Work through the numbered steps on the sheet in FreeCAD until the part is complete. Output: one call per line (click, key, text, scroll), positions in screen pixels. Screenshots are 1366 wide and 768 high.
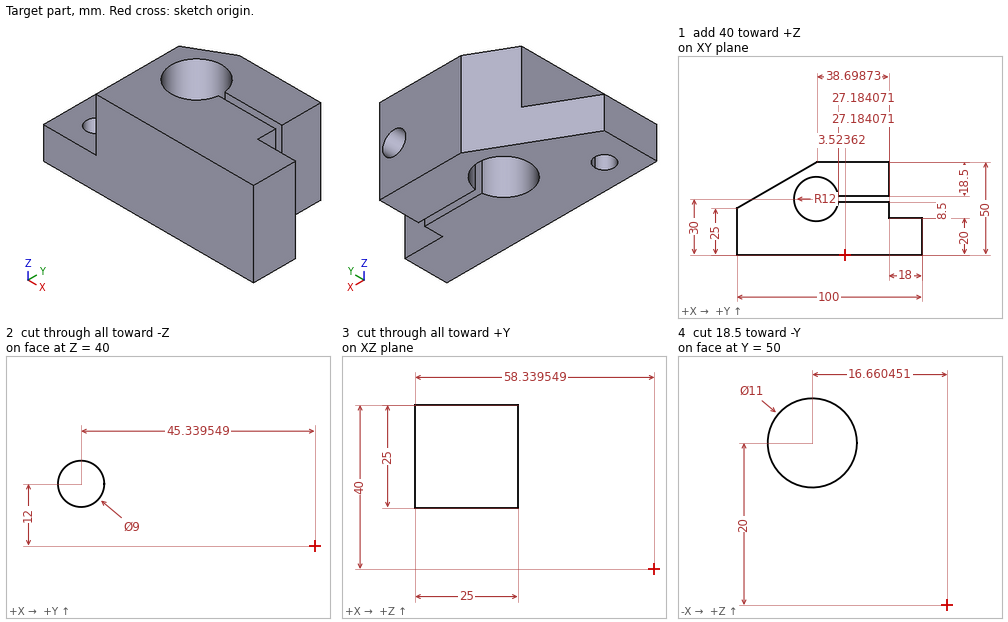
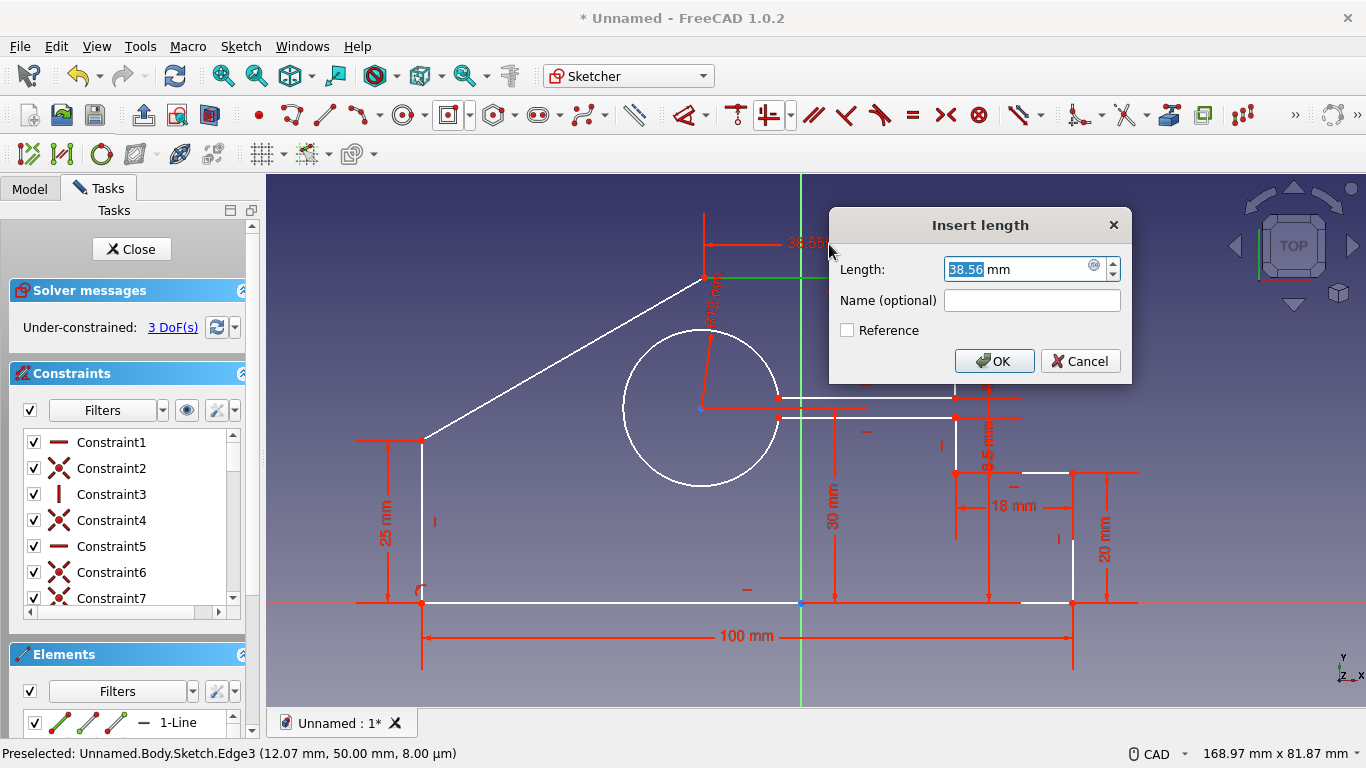
text(38.69873)
key(Return)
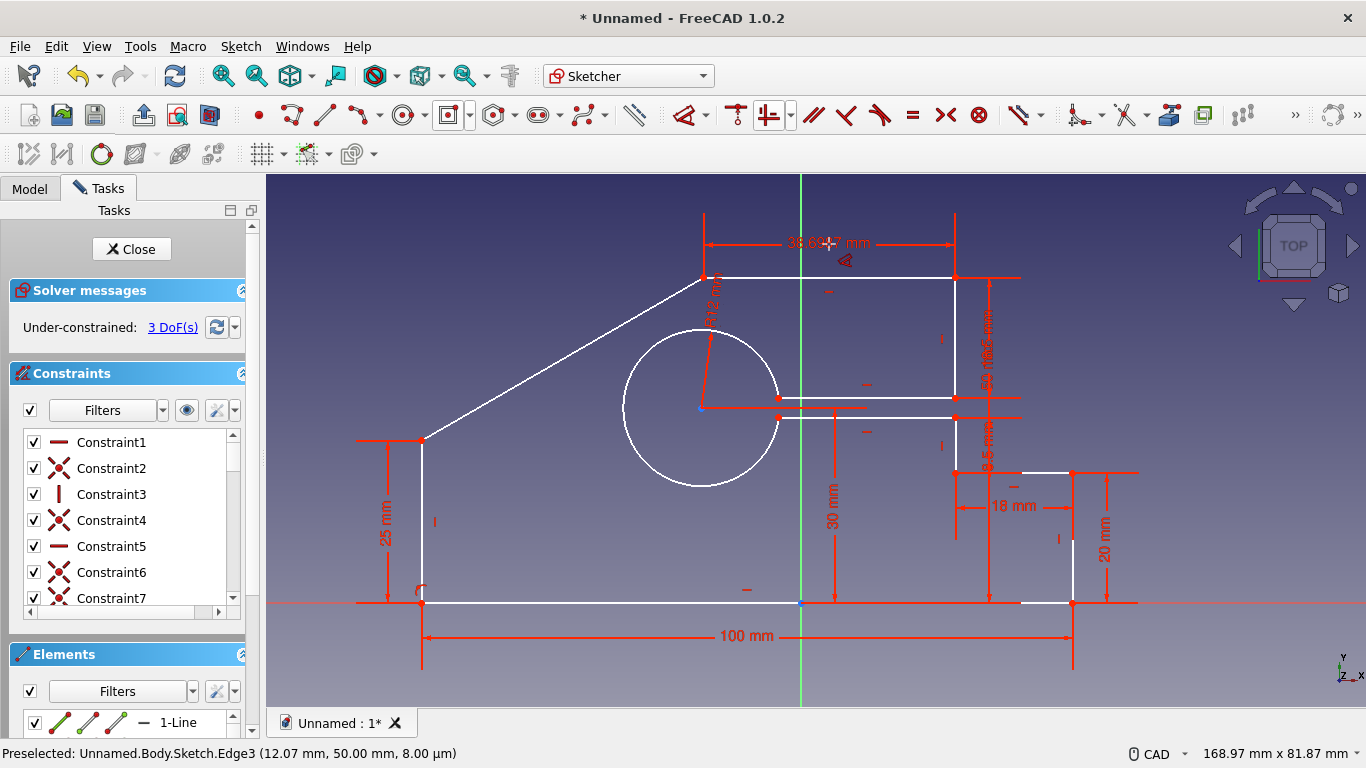
scroll(779, 398, up, 3)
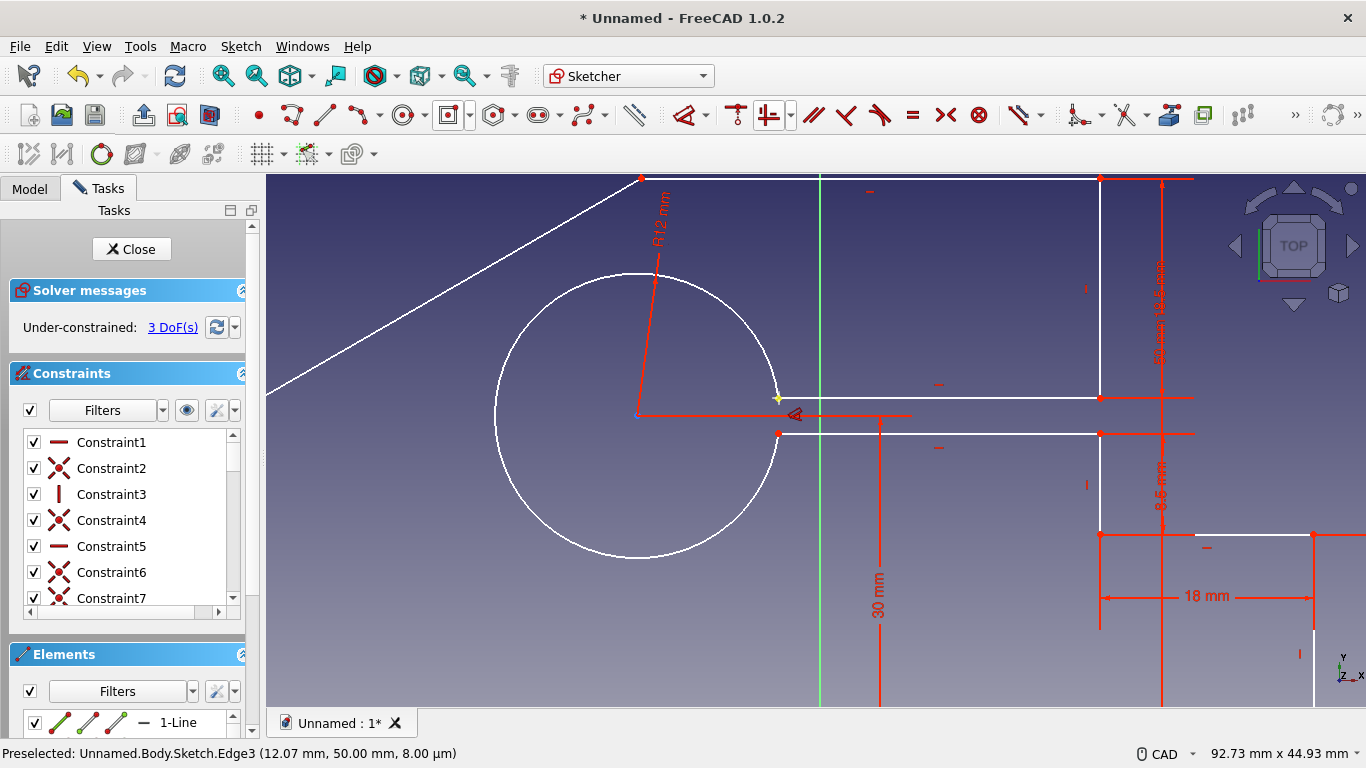
click(778, 398)
click(799, 364)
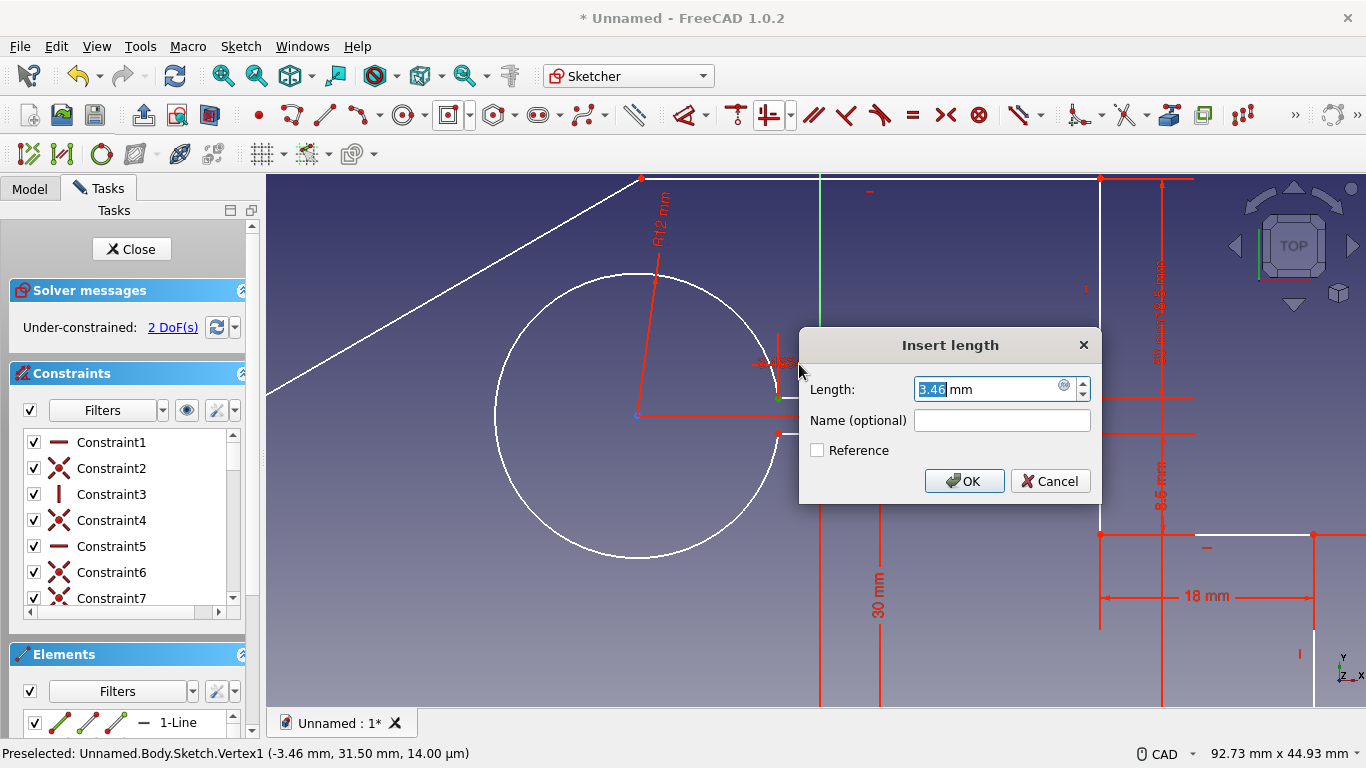
text(3.52362)
key(Return)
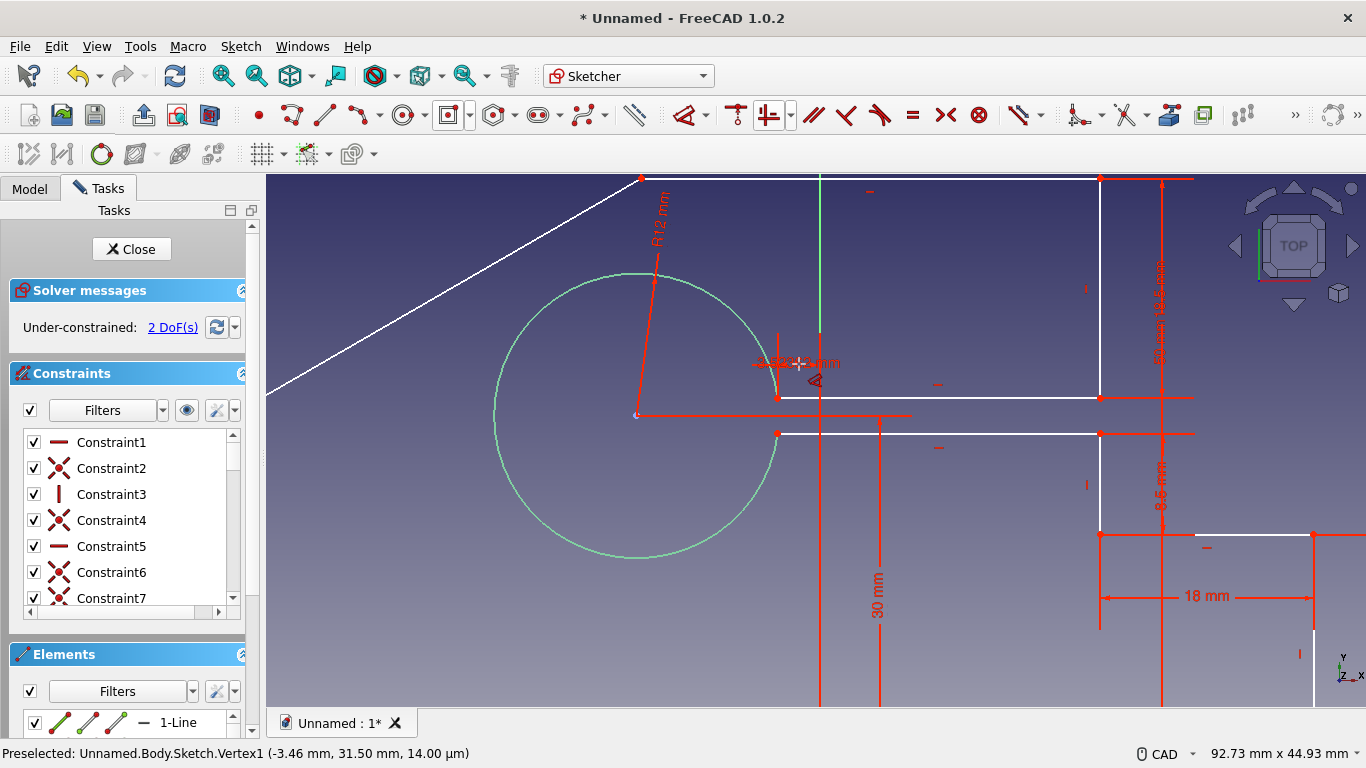
click(874, 398)
click(939, 364)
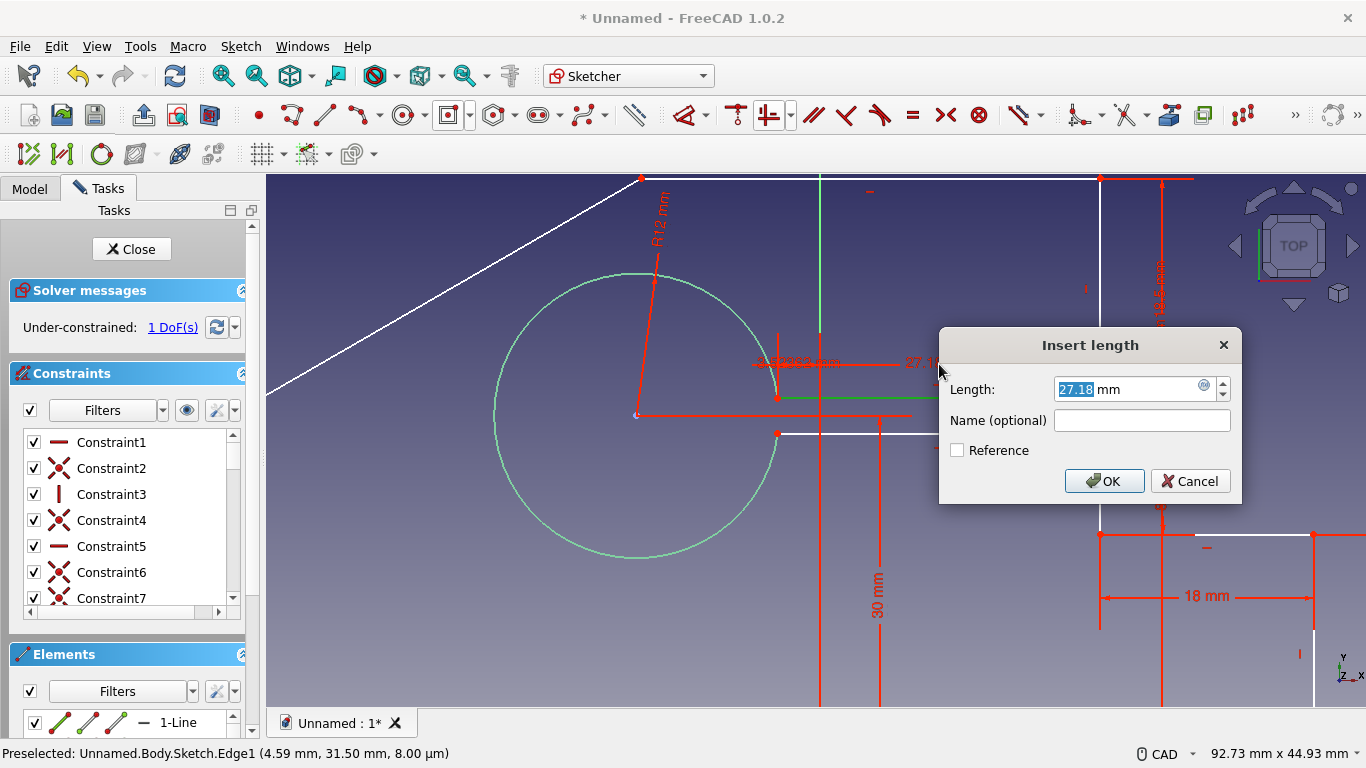
text(27.184071)
key(Return)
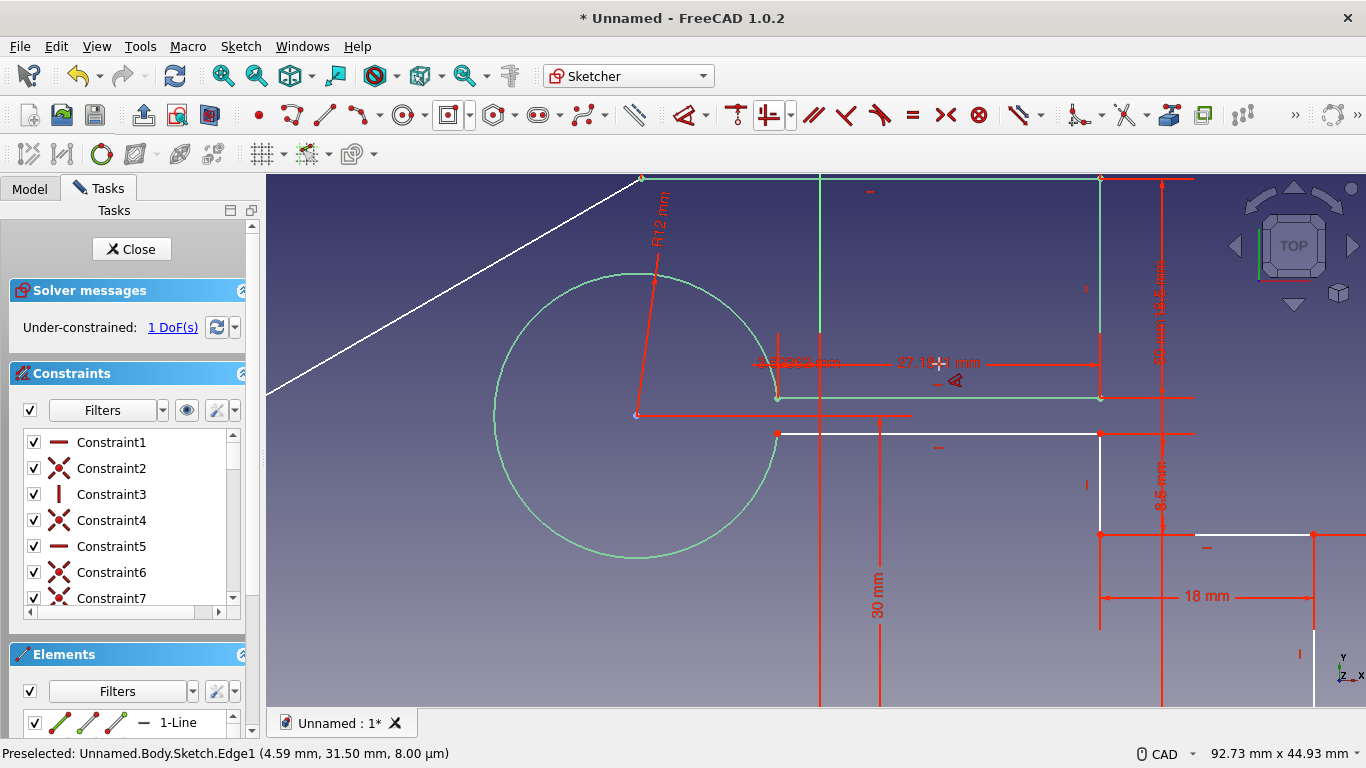
click(1004, 434)
click(939, 468)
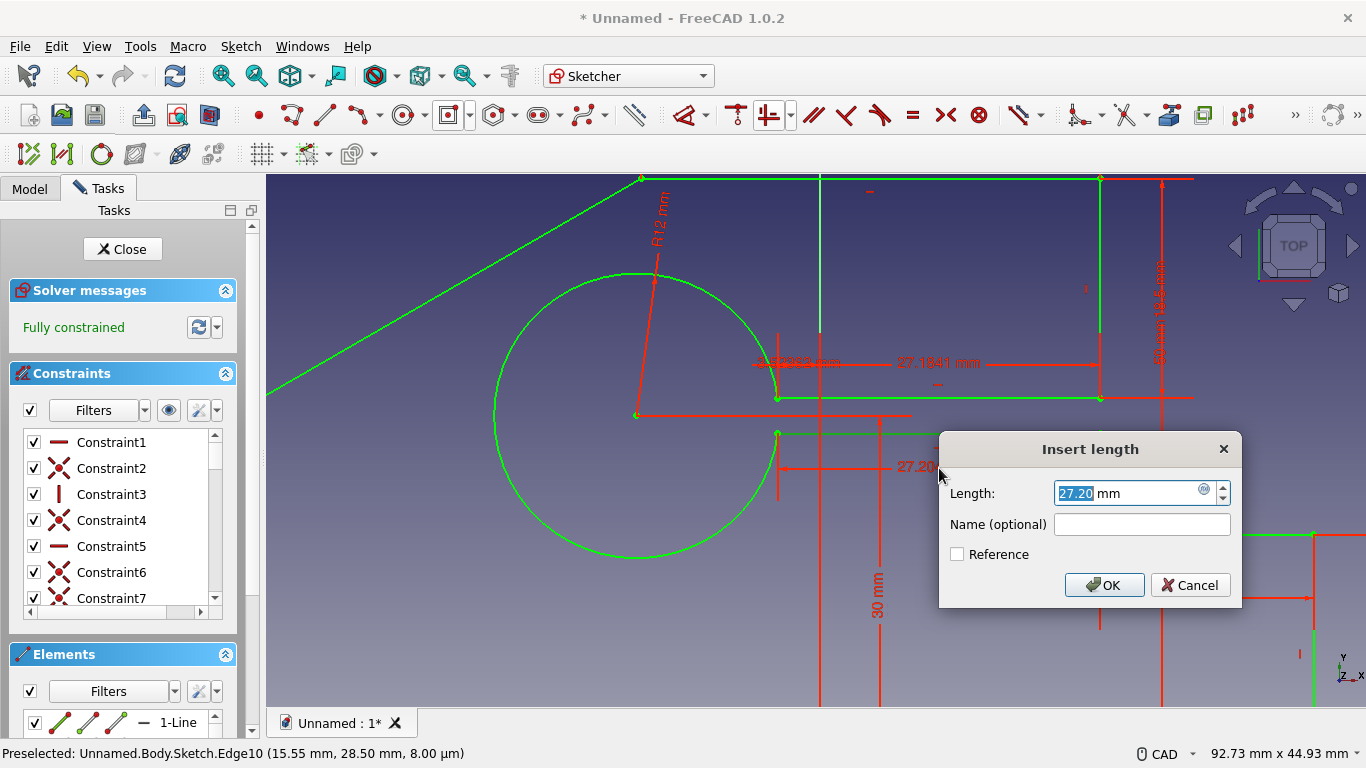
text(27.184071)
key(Return)
key(Escape)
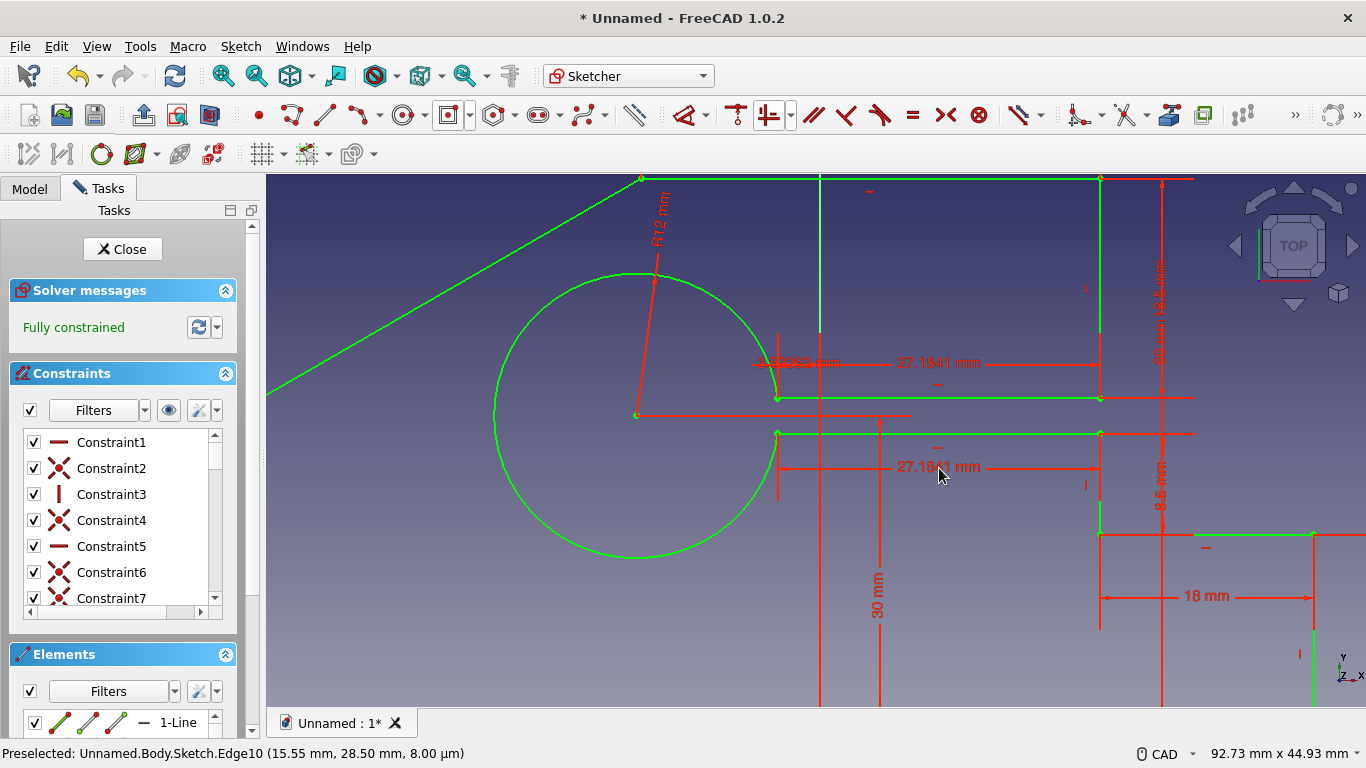
click(123, 249)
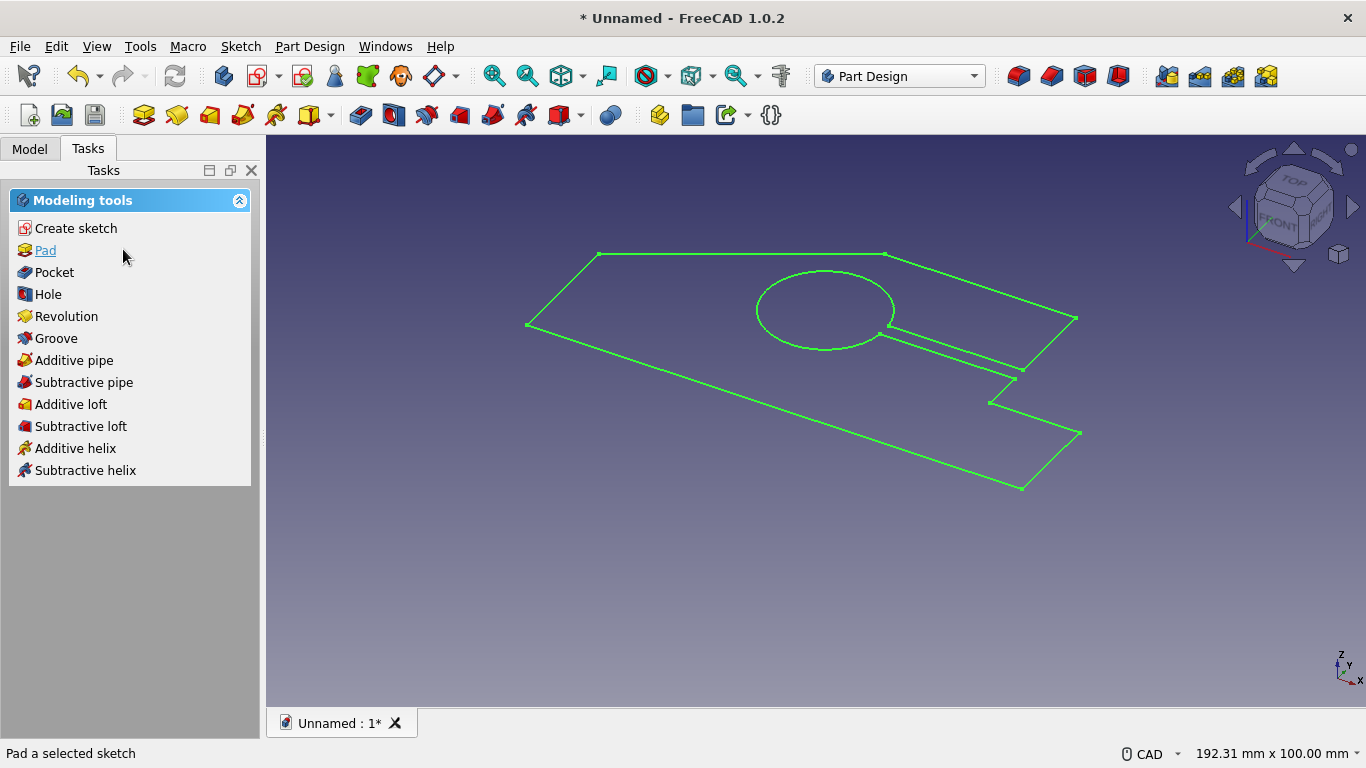
click(144, 116)